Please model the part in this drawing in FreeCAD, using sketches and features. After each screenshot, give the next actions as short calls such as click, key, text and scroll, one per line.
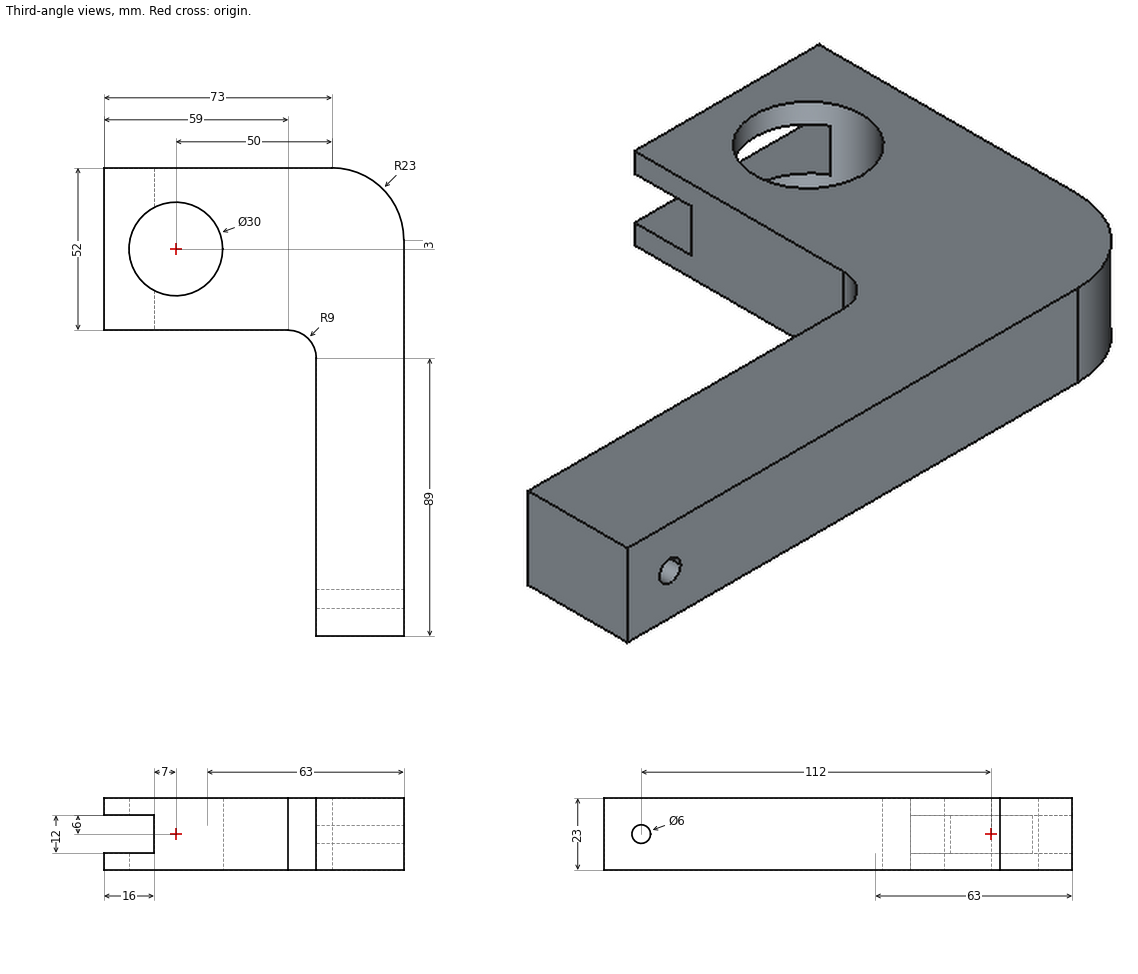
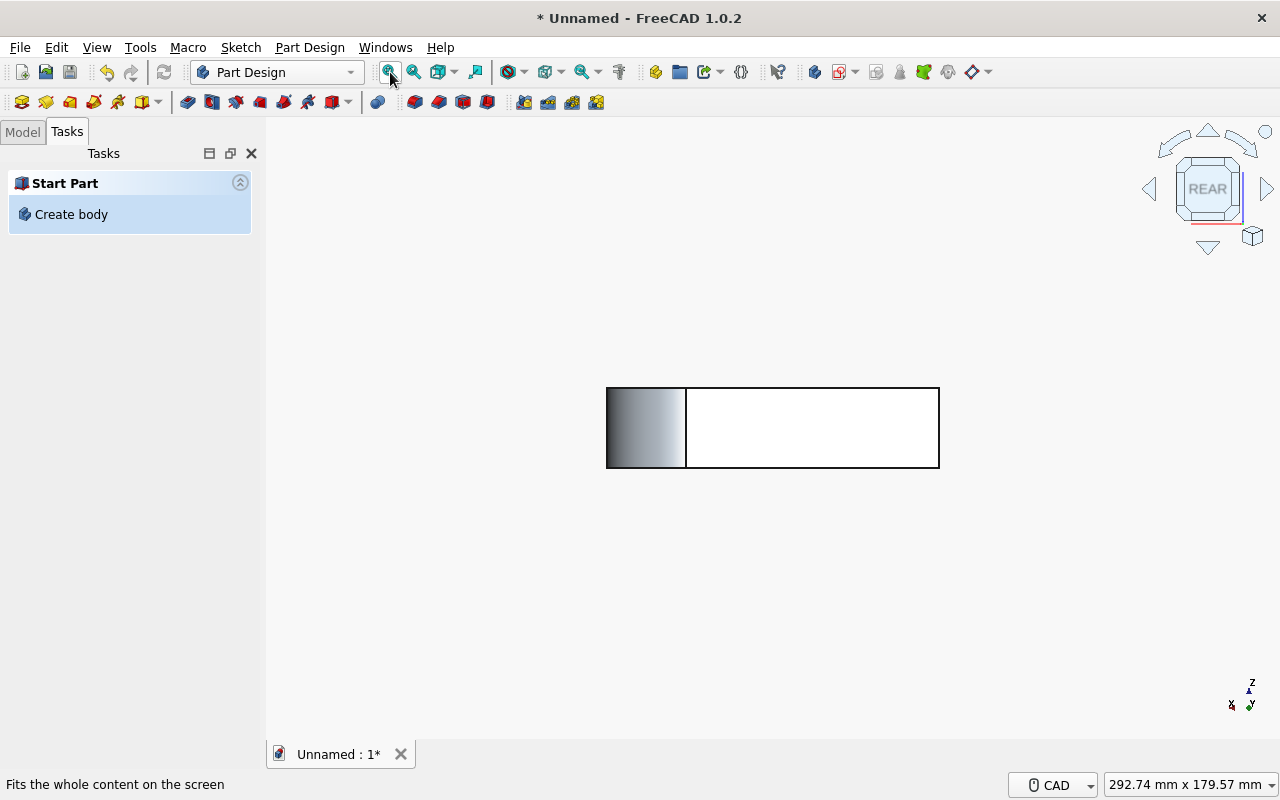
click(741, 427)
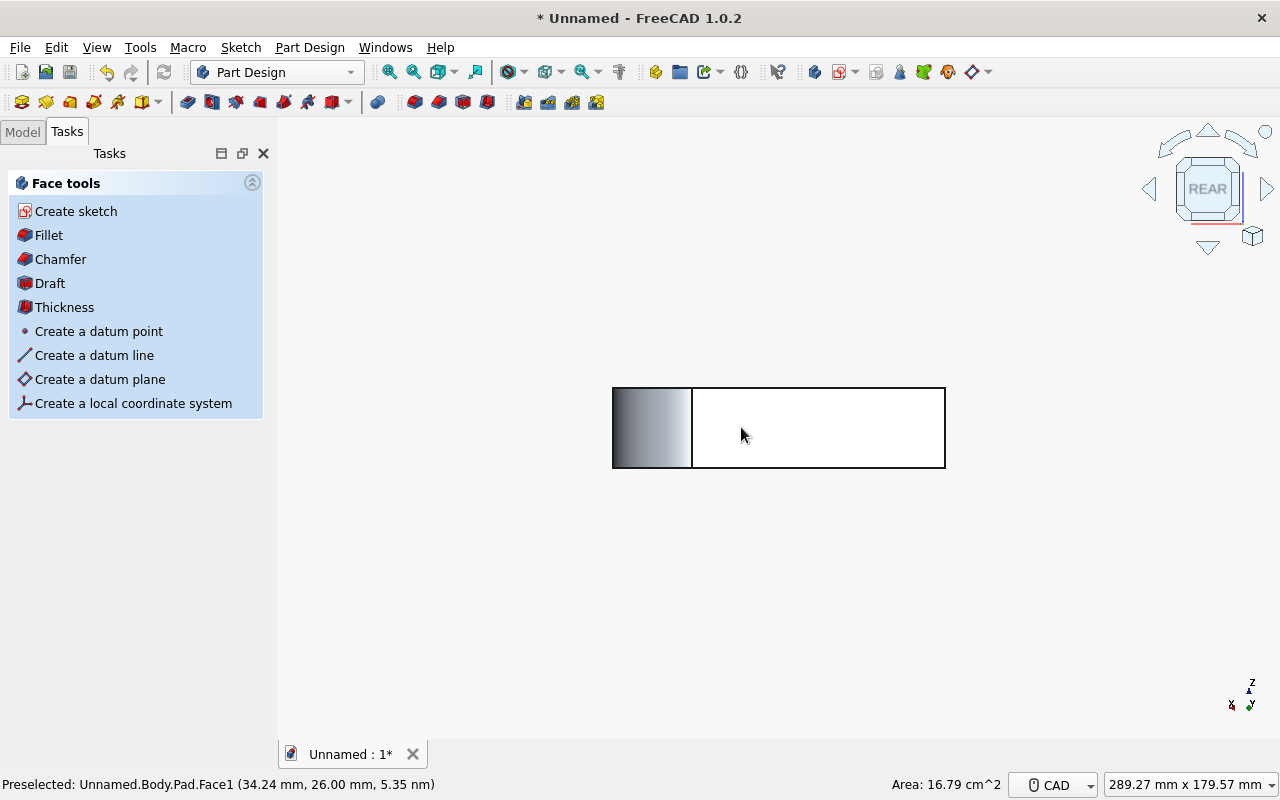
click(840, 72)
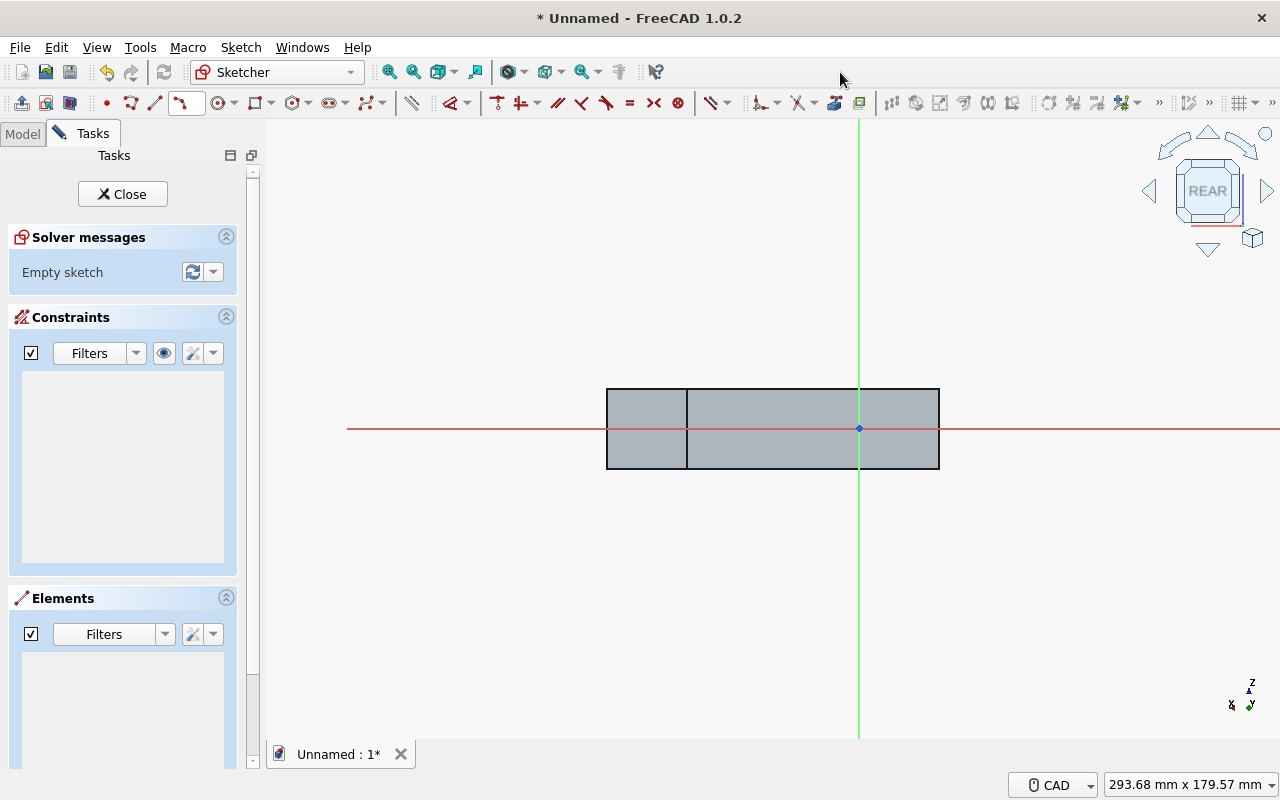
scroll(929, 429, up, 10)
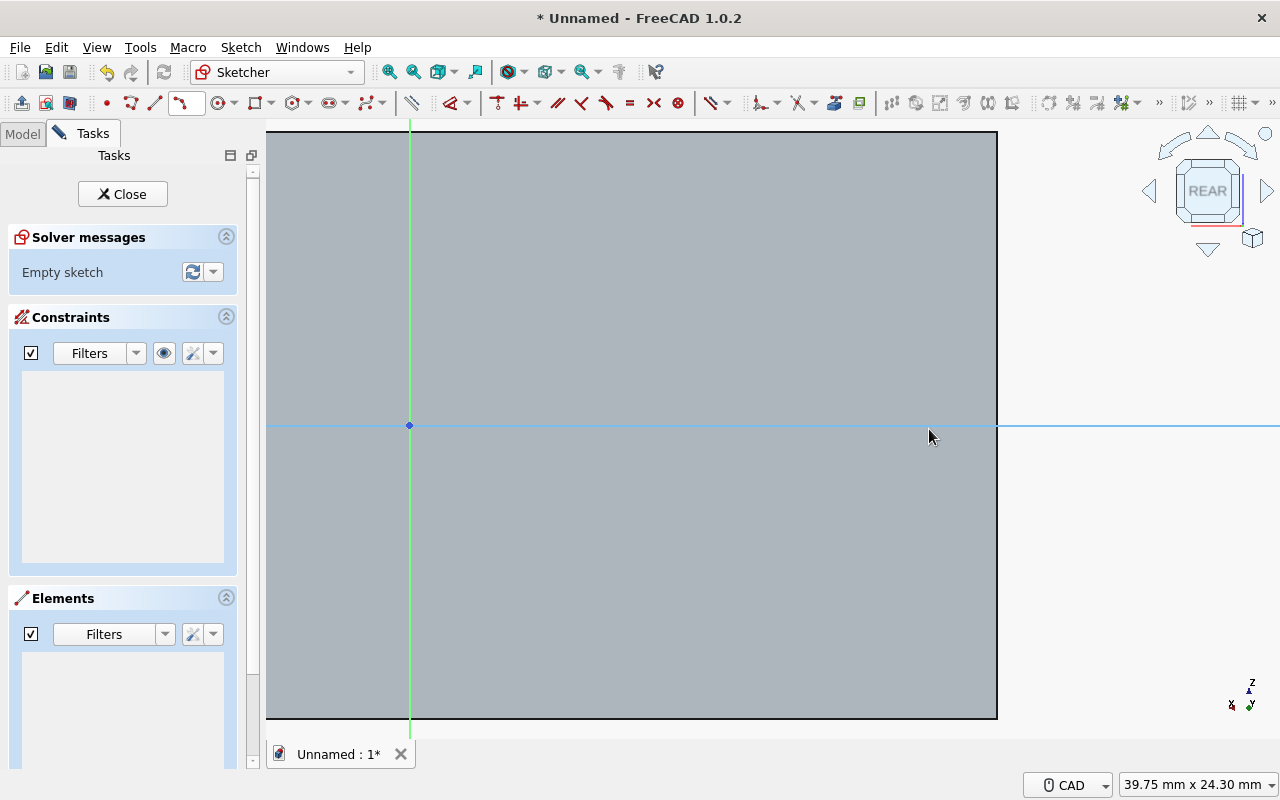
click(256, 104)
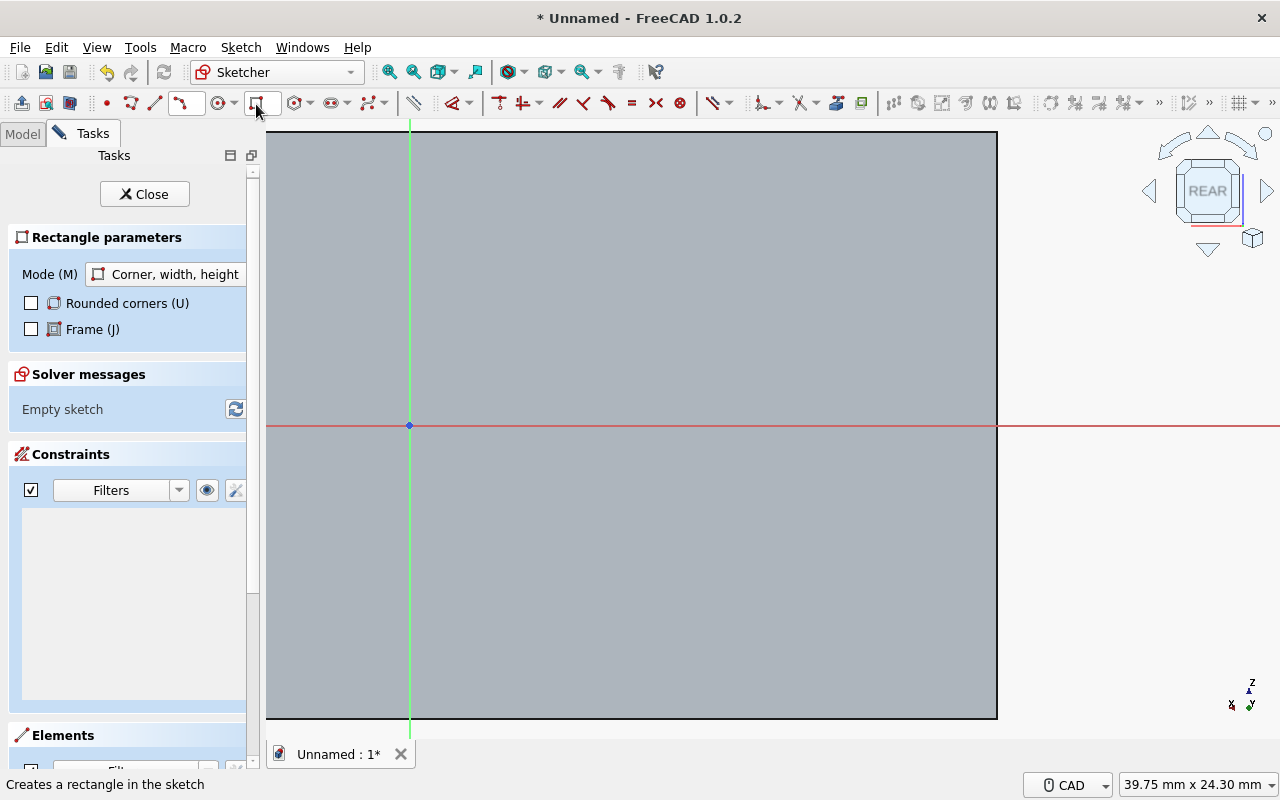
click(589, 273)
move(997, 579)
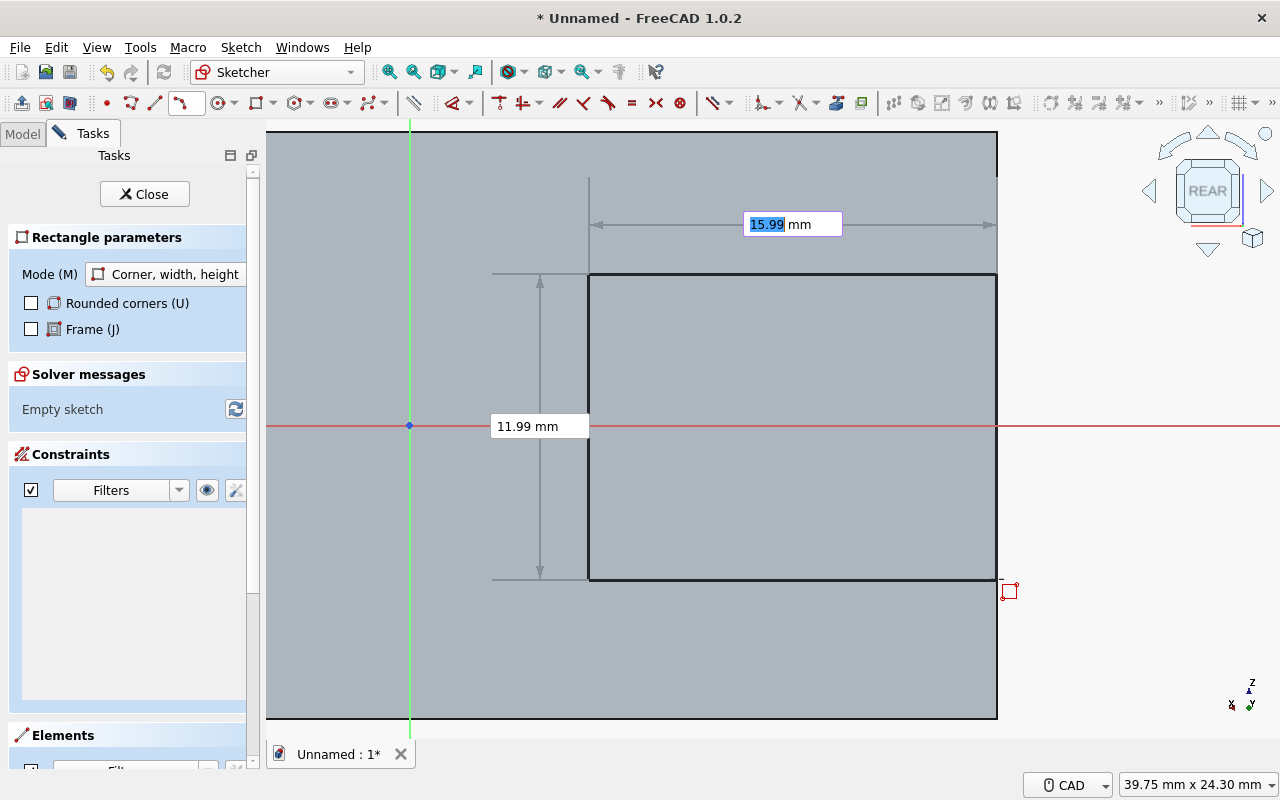
text(16)
key(Tab)
text(12)
key(Return)
key(Escape)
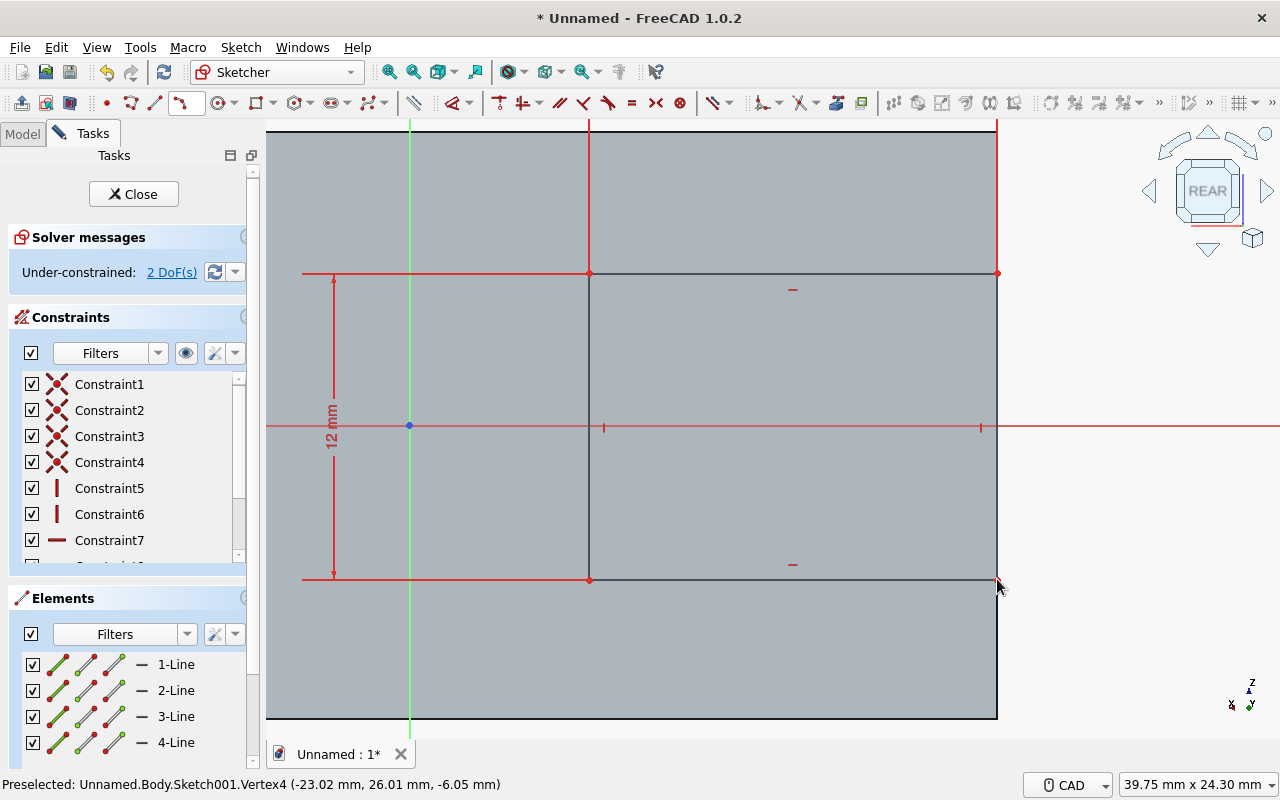
click(452, 104)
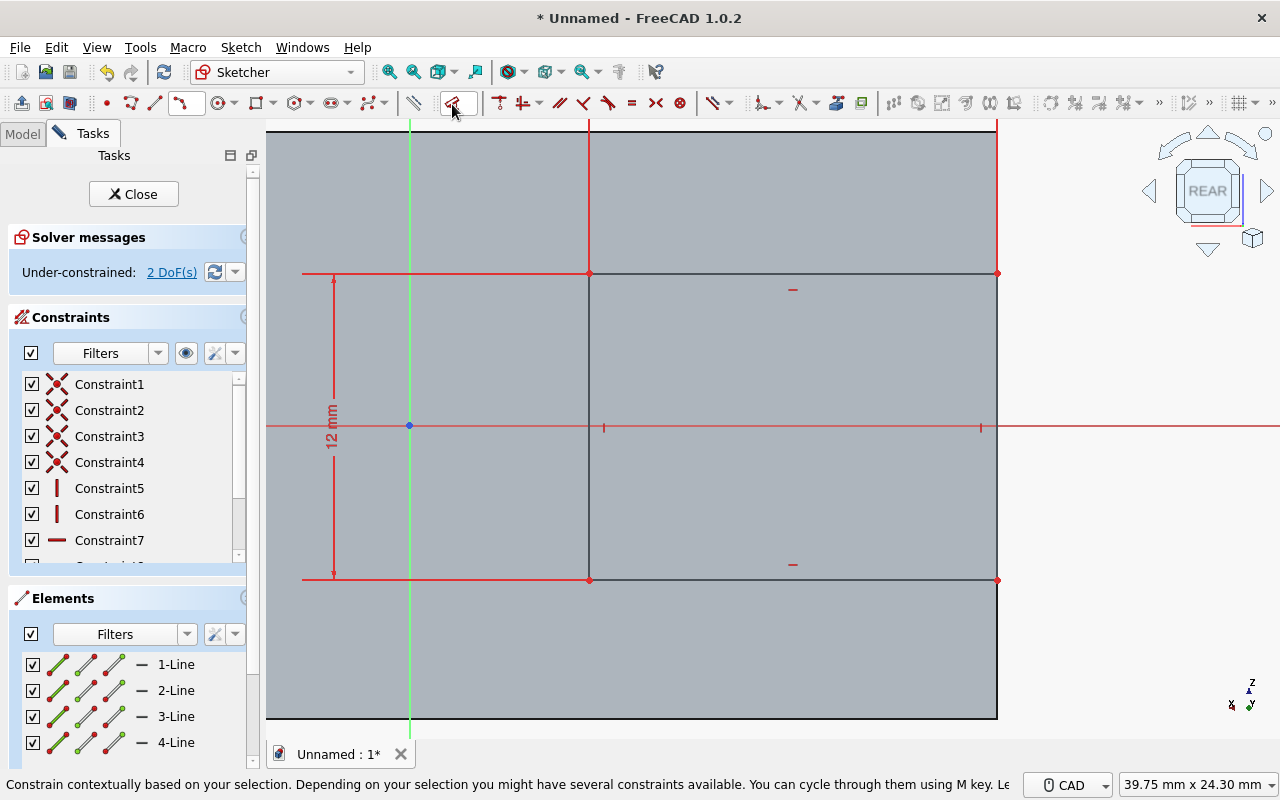
click(589, 274)
click(499, 240)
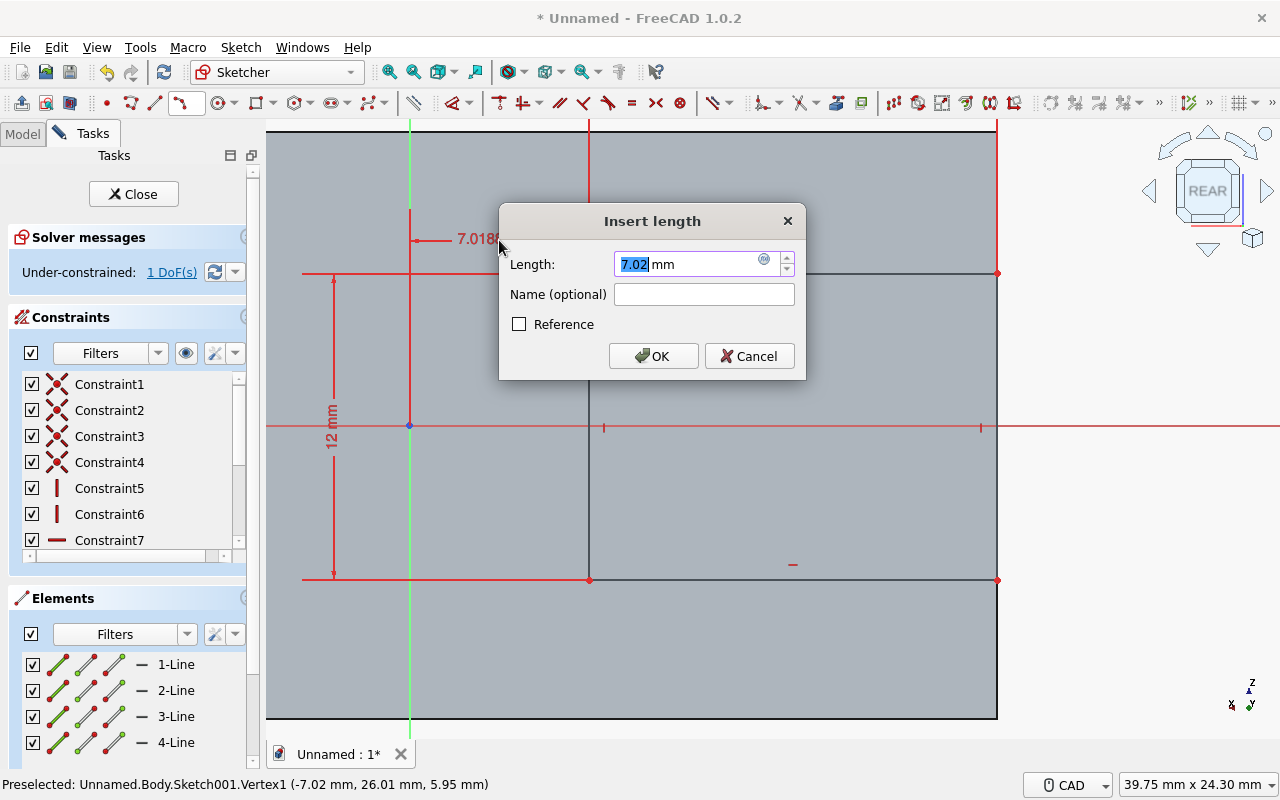
text(7)
key(Return)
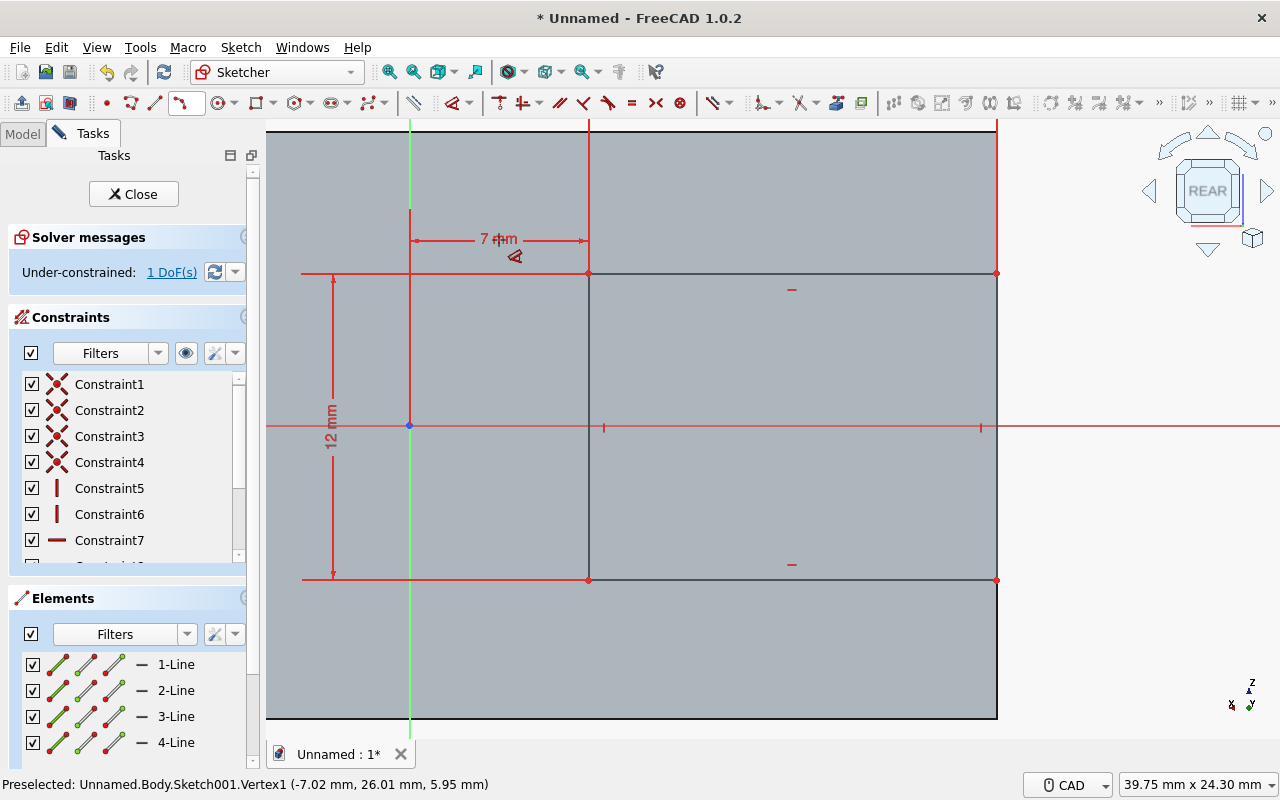
click(589, 274)
click(376, 350)